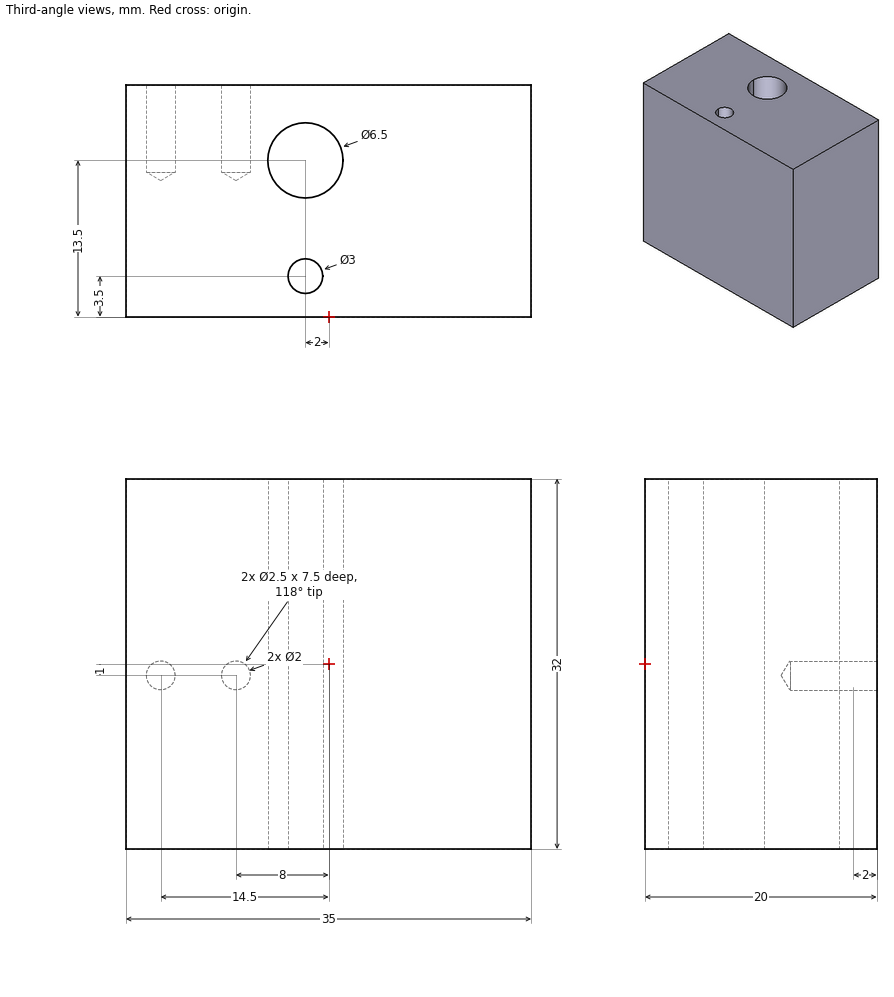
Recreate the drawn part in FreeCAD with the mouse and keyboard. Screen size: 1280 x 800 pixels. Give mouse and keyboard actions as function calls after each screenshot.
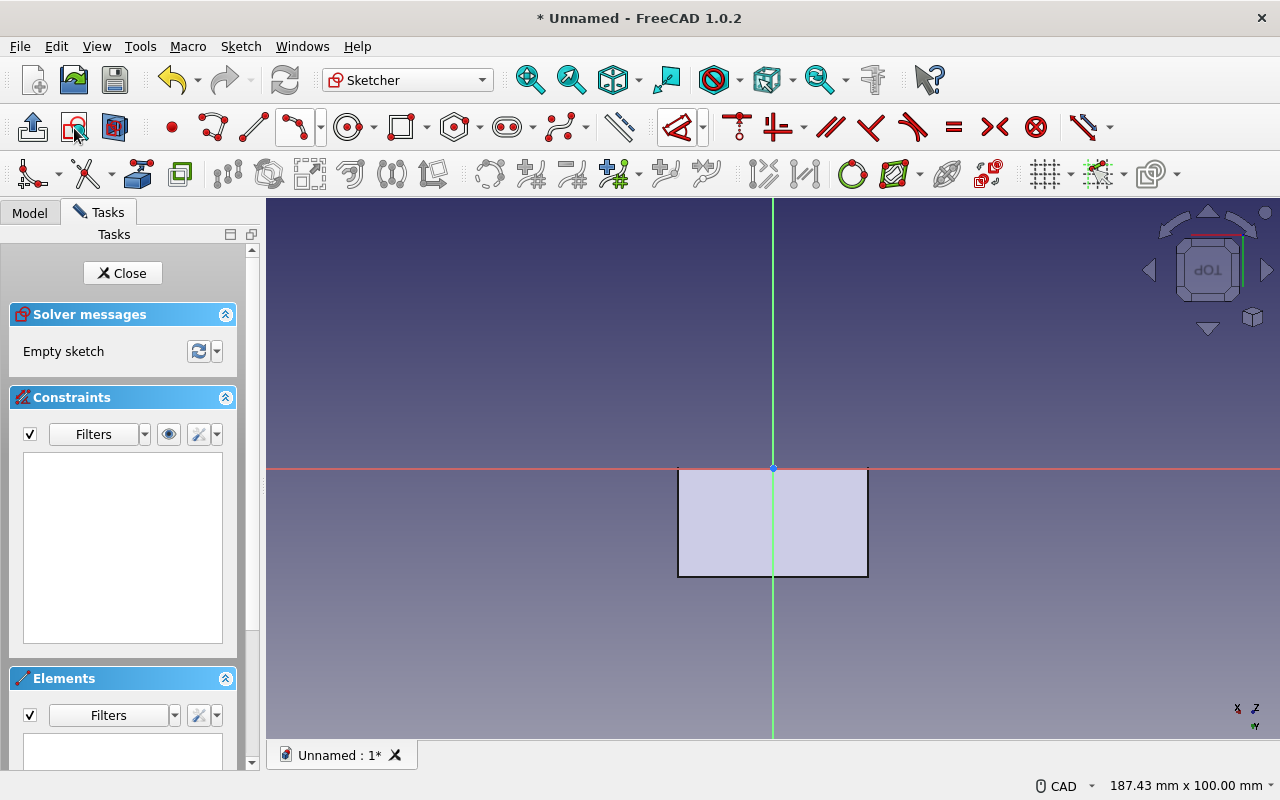
scroll(794, 551, up, 11)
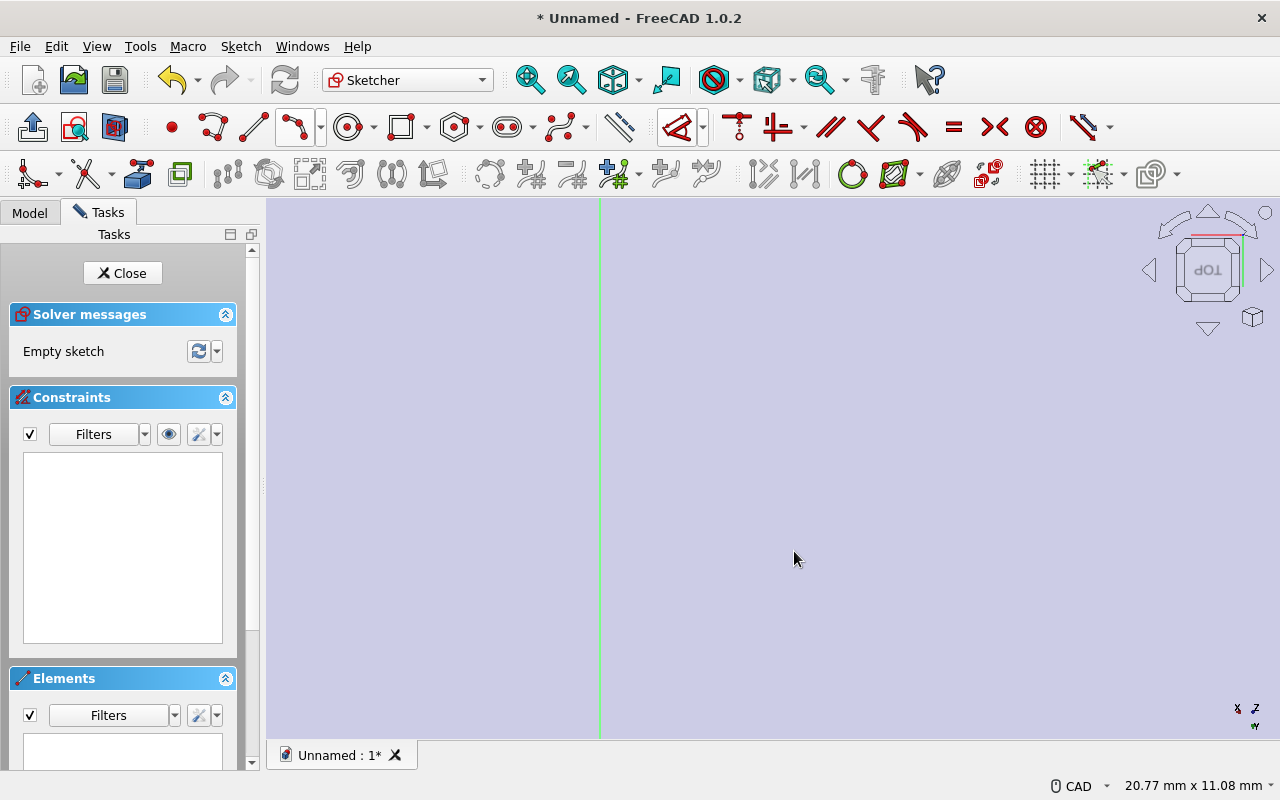
key(g)
key(c)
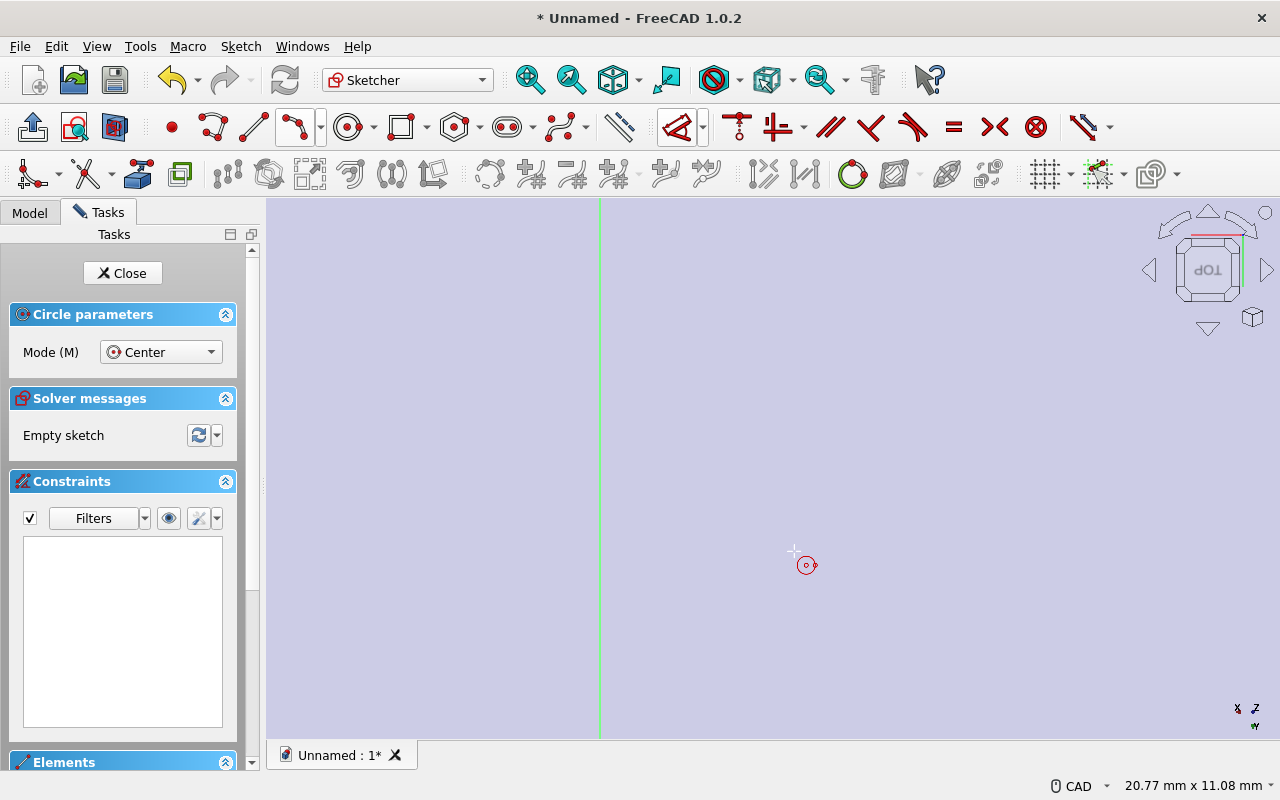
click(698, 460)
click(810, 348)
key(Escape)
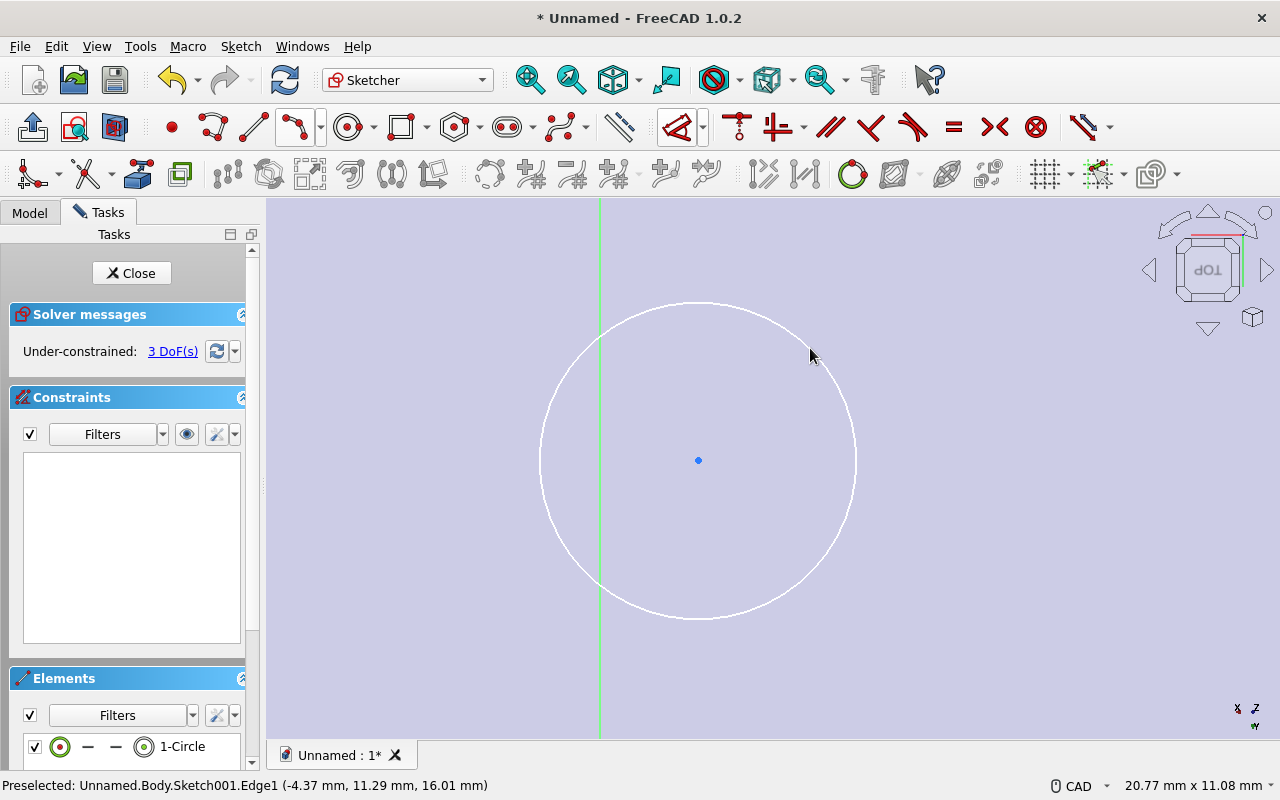
click(810, 349)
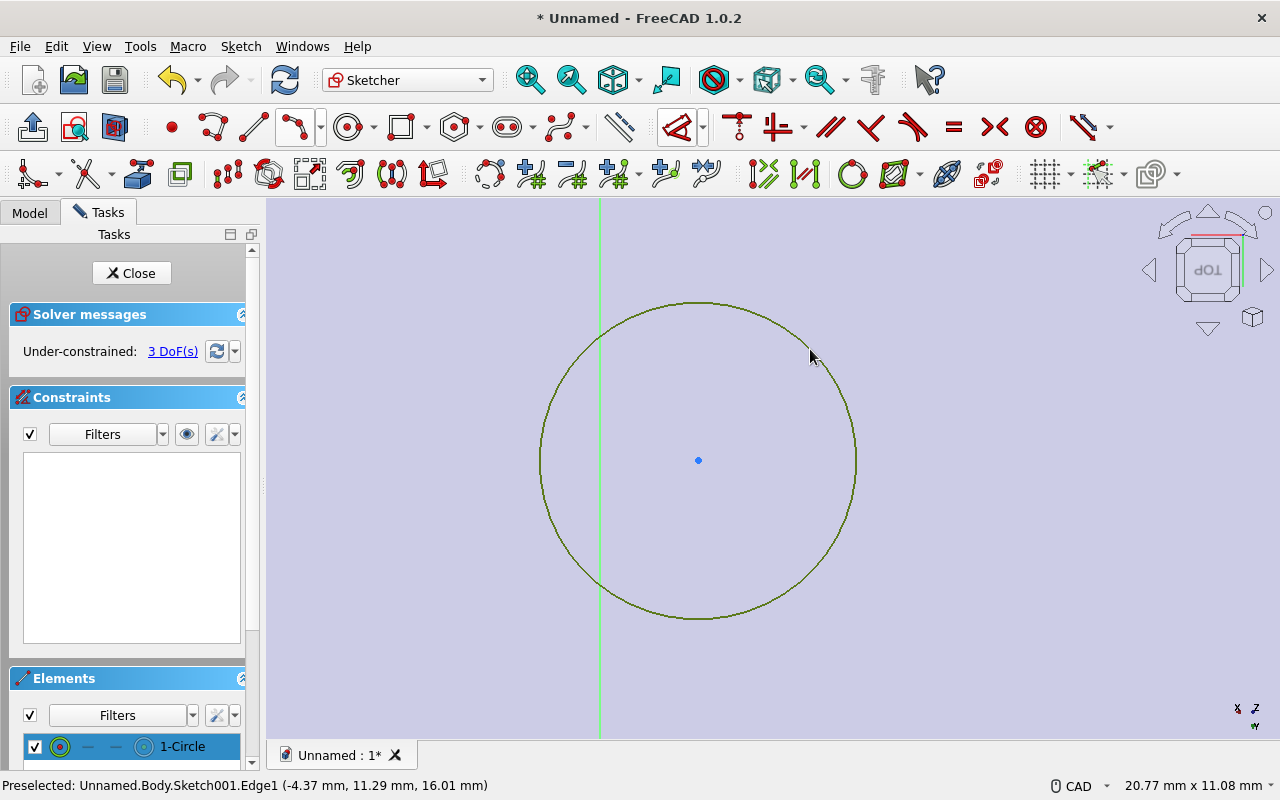
key(k)
key(o)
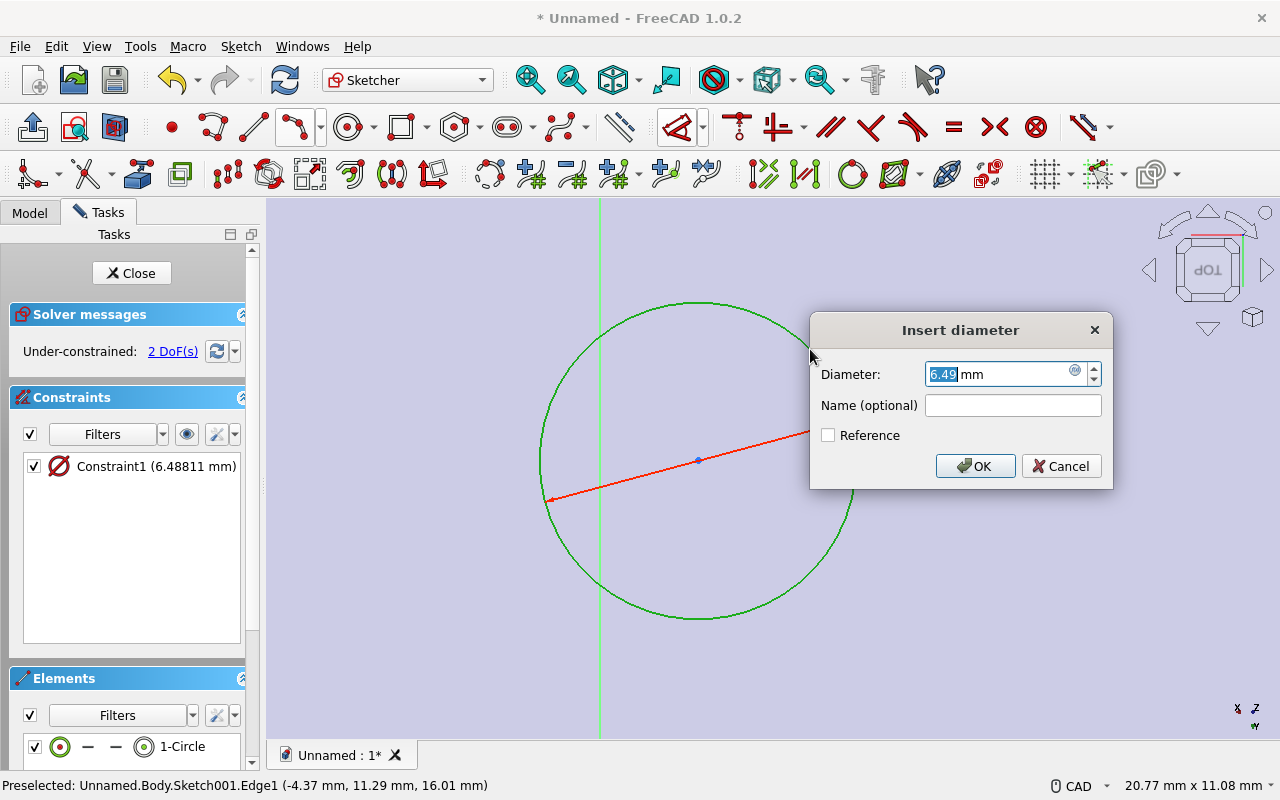
text(6.5)
key(Return)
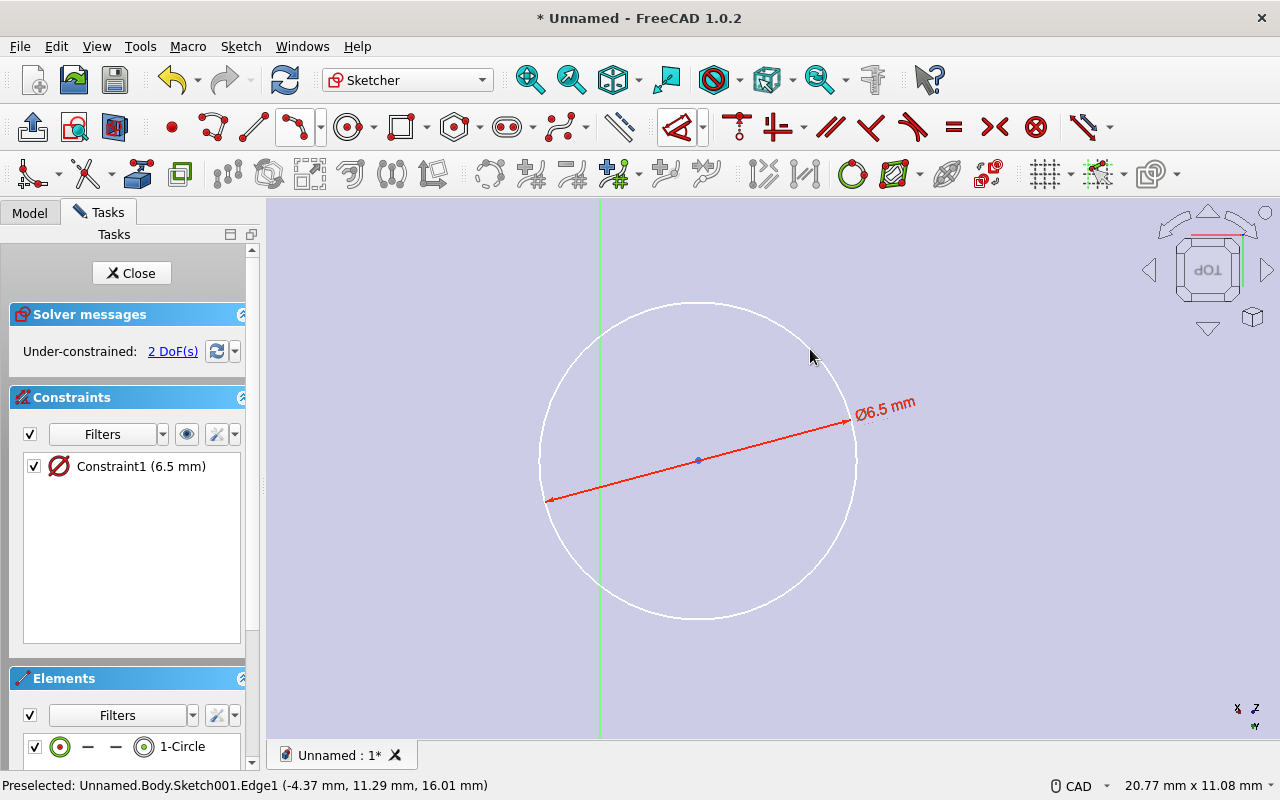
click(698, 461)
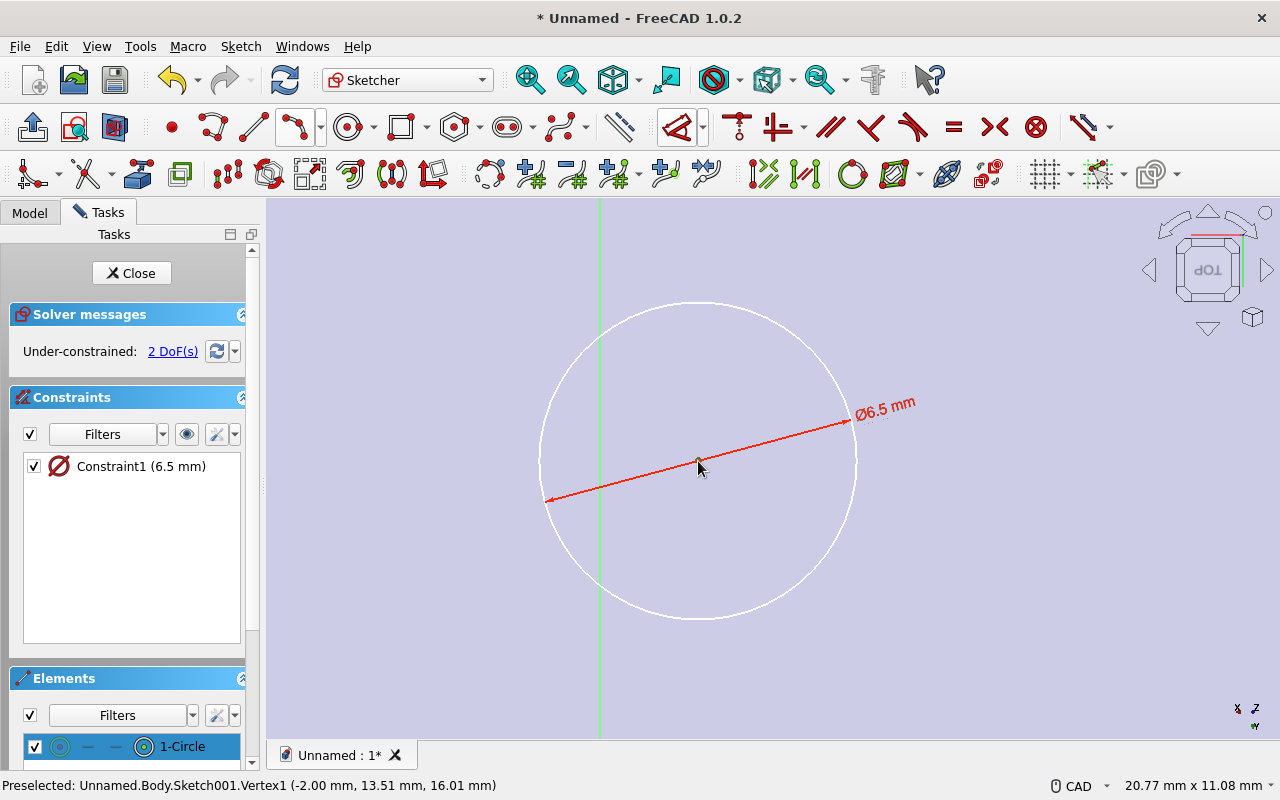
key(l)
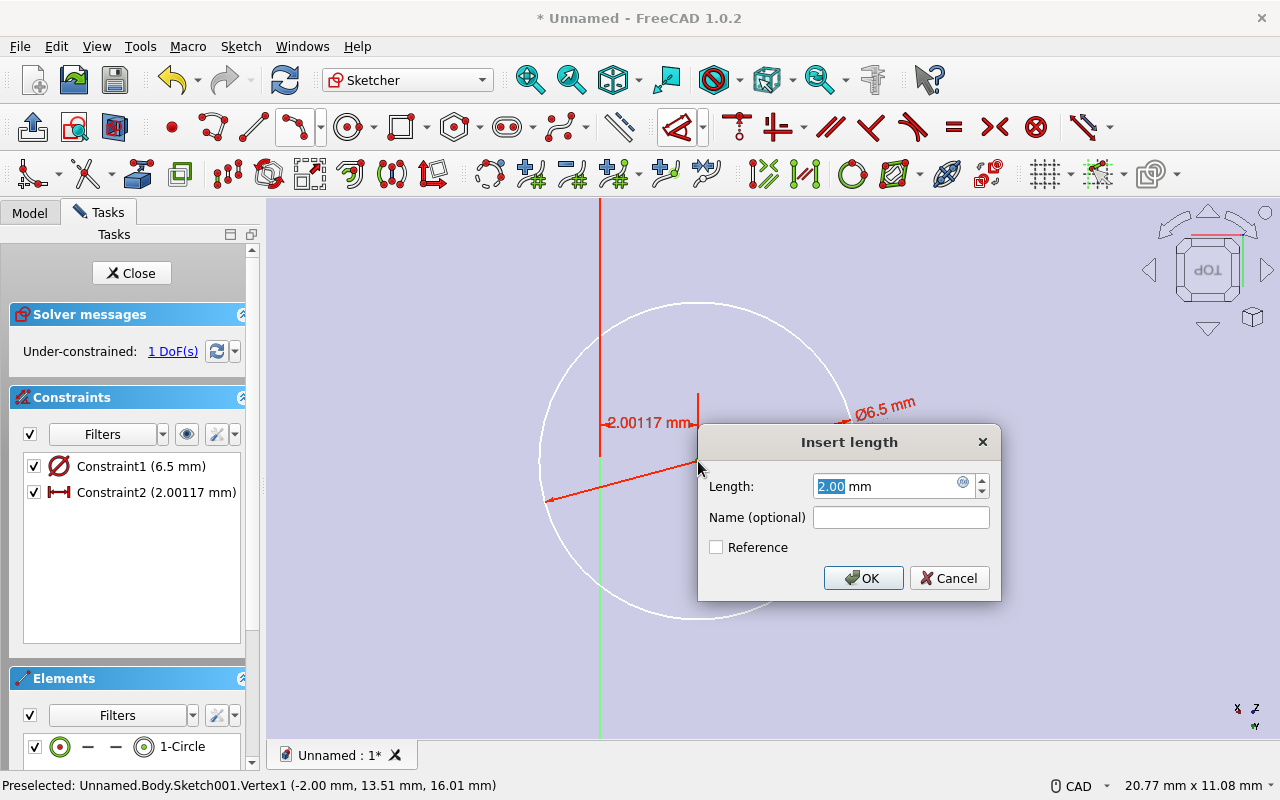
text(2)
key(Return)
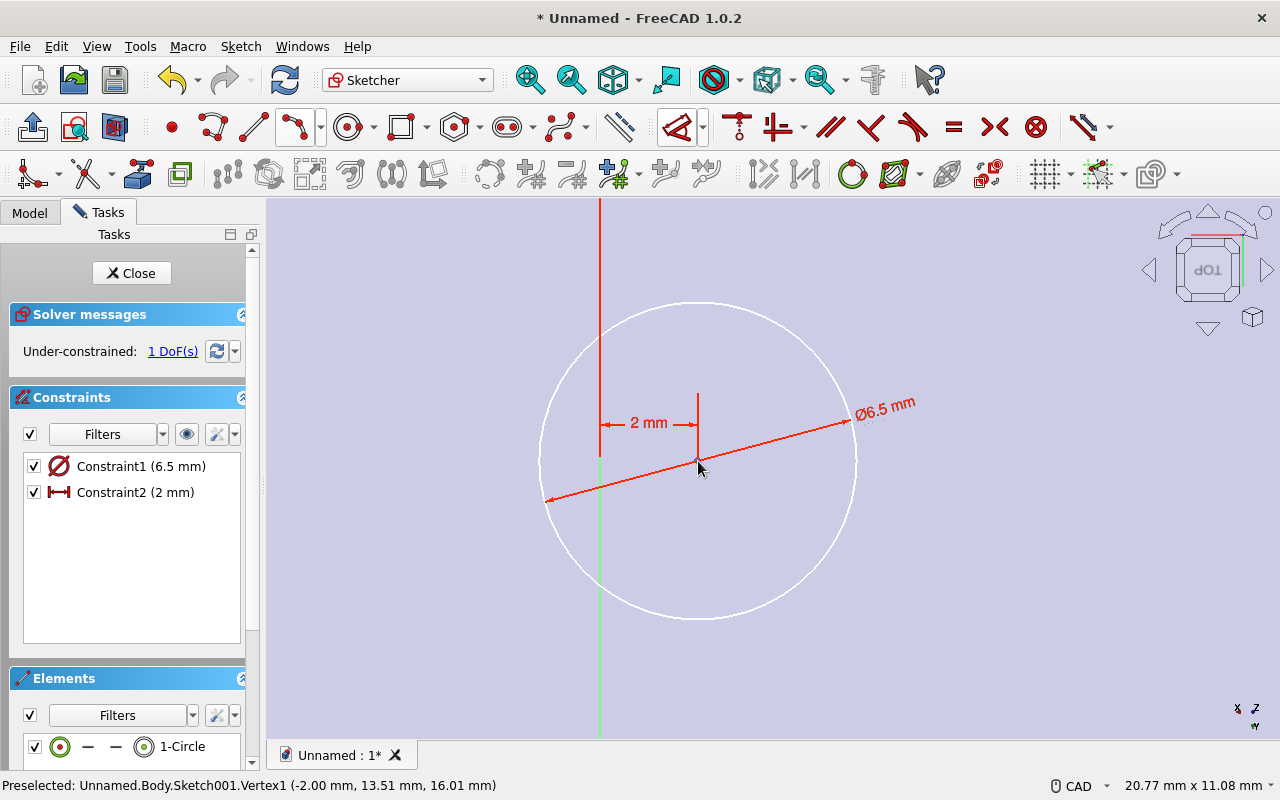
click(698, 461)